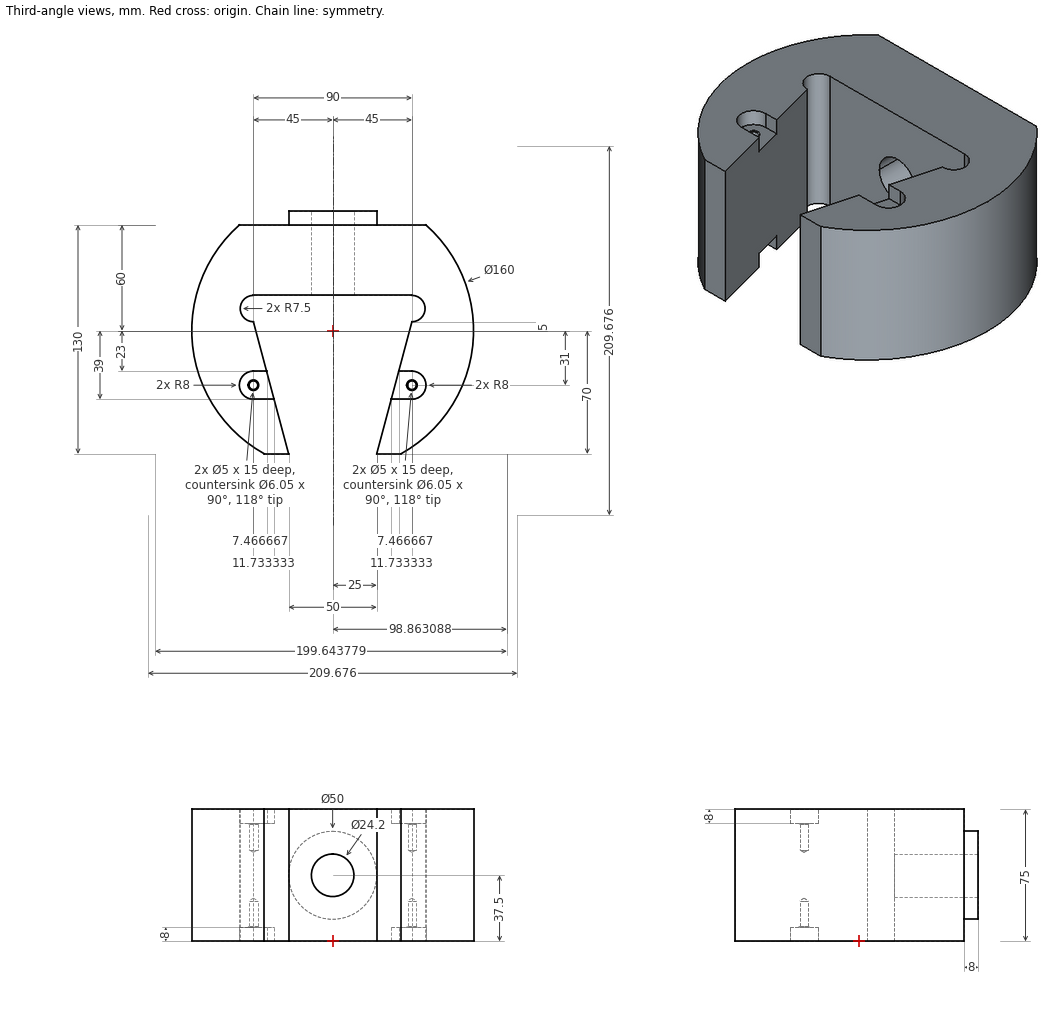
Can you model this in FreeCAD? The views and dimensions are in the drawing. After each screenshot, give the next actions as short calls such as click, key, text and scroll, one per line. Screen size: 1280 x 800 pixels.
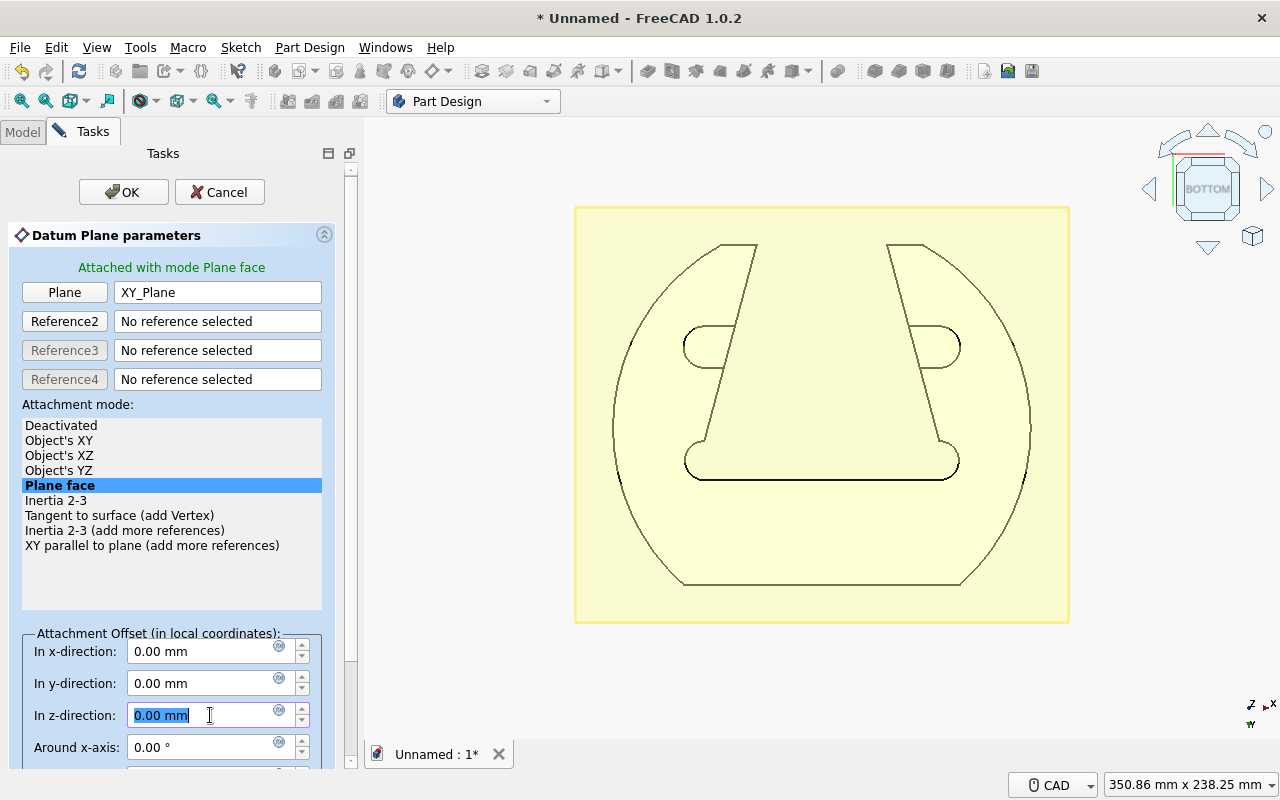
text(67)
key(Tab)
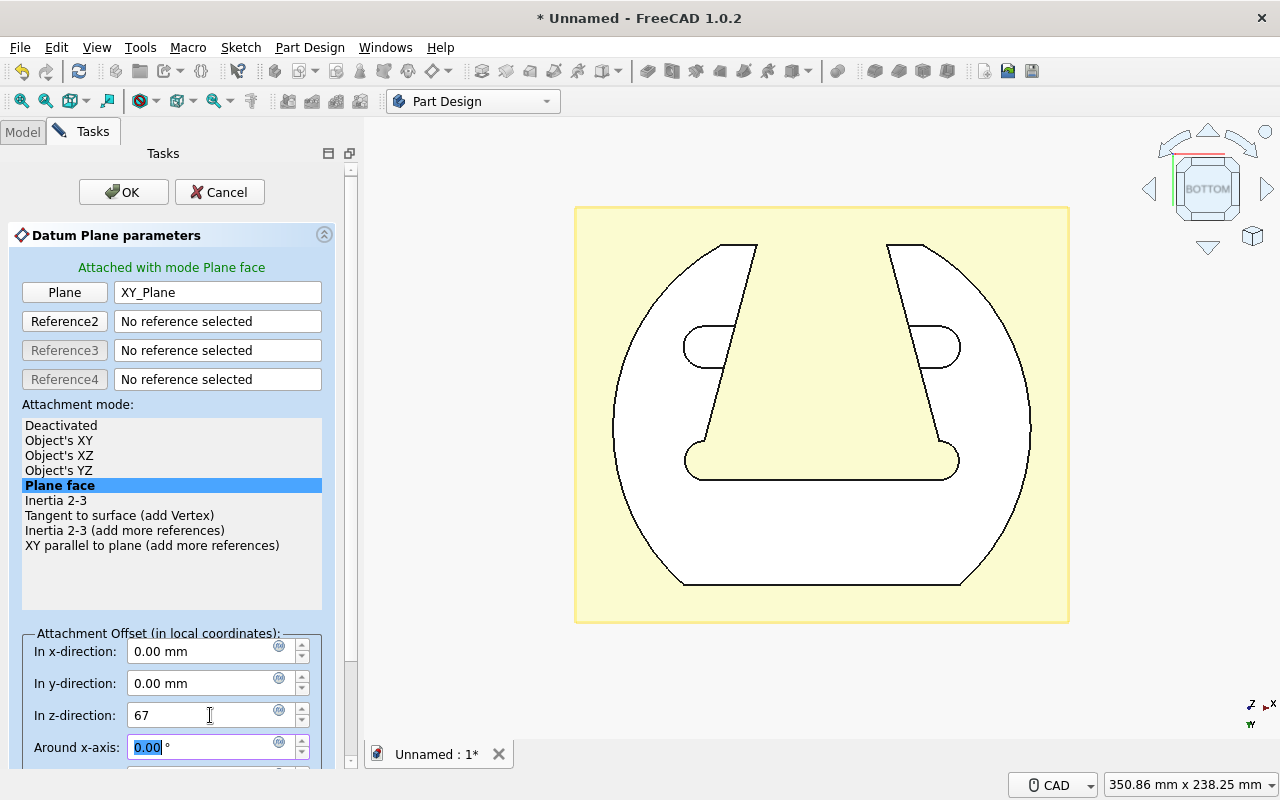
click(124, 192)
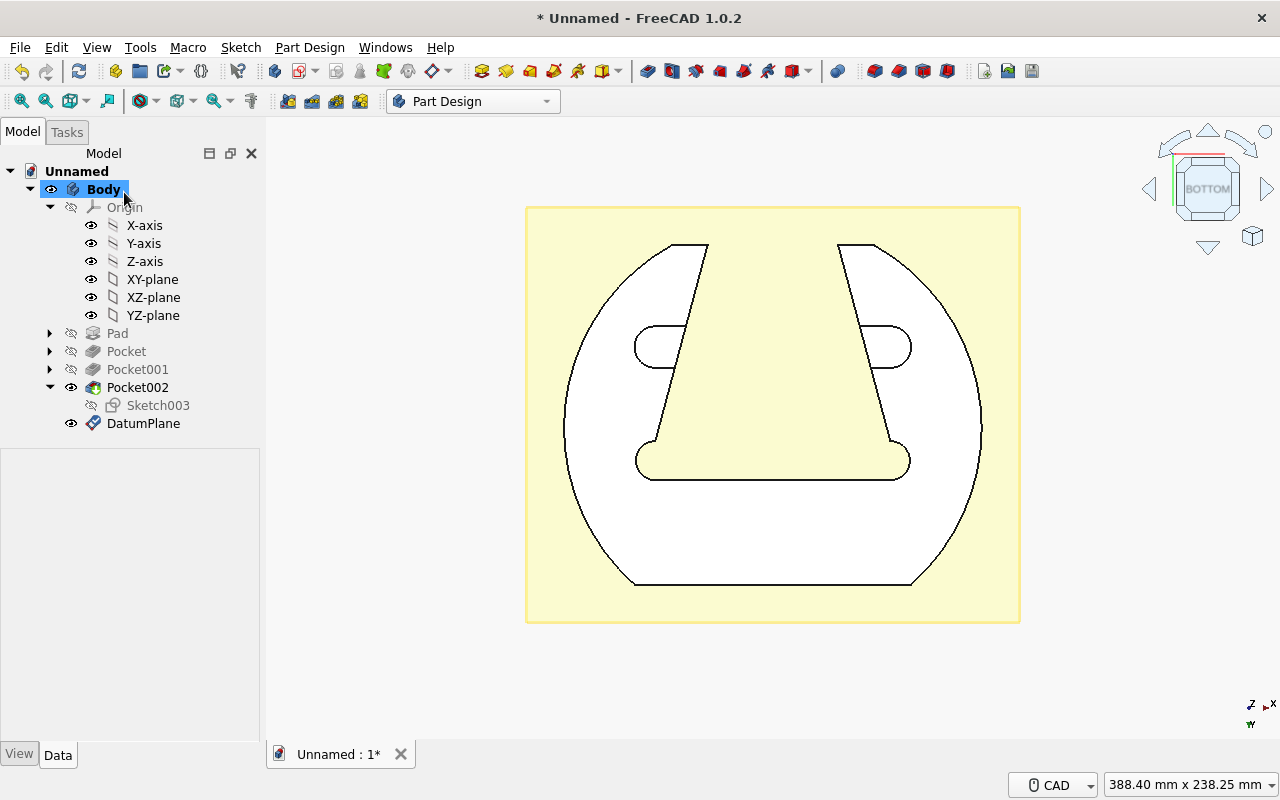
click(116, 423)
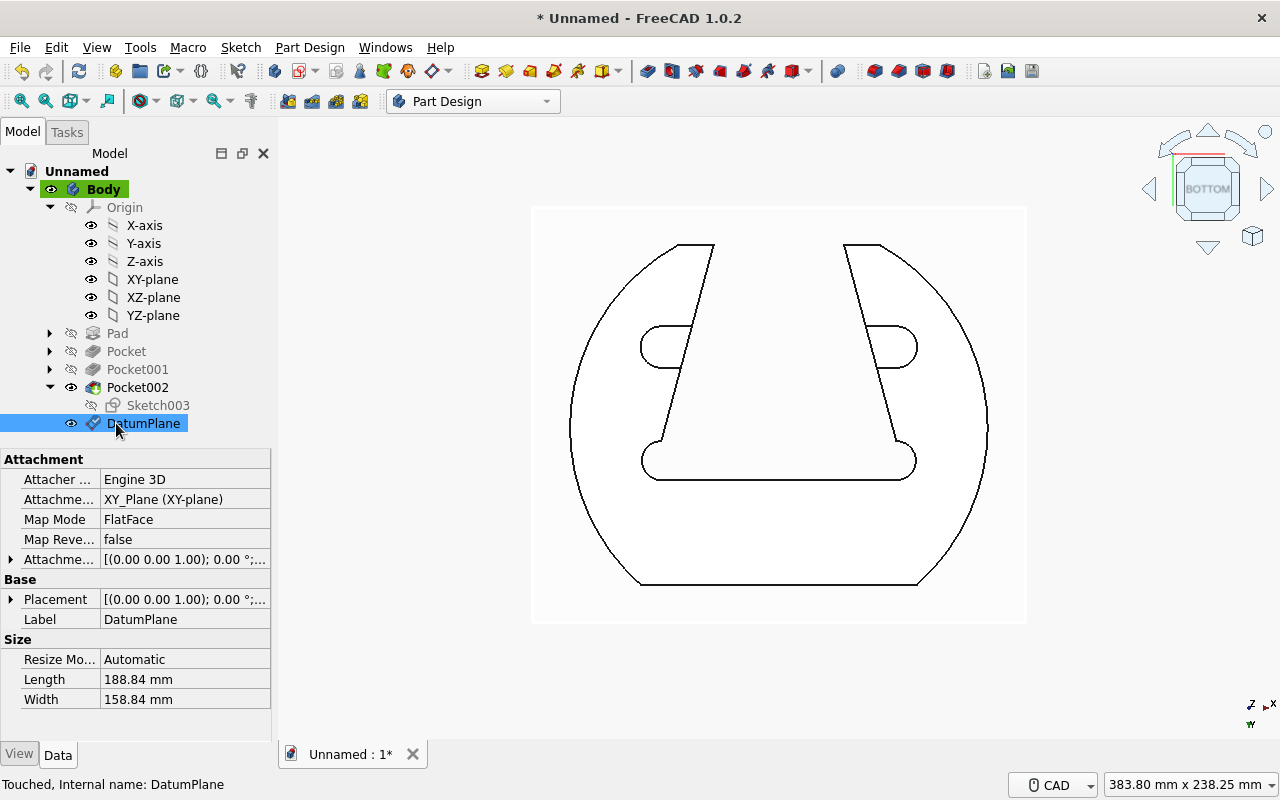
click(300, 72)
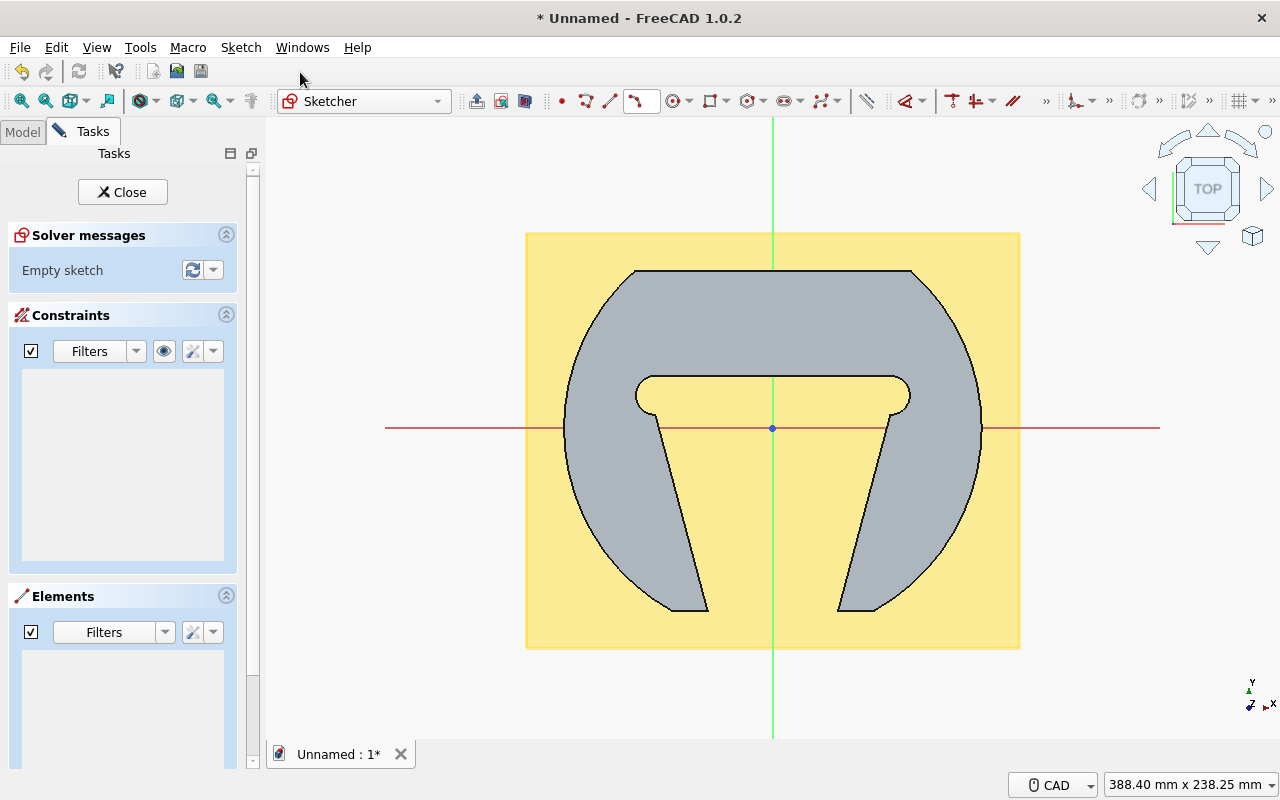
click(526, 102)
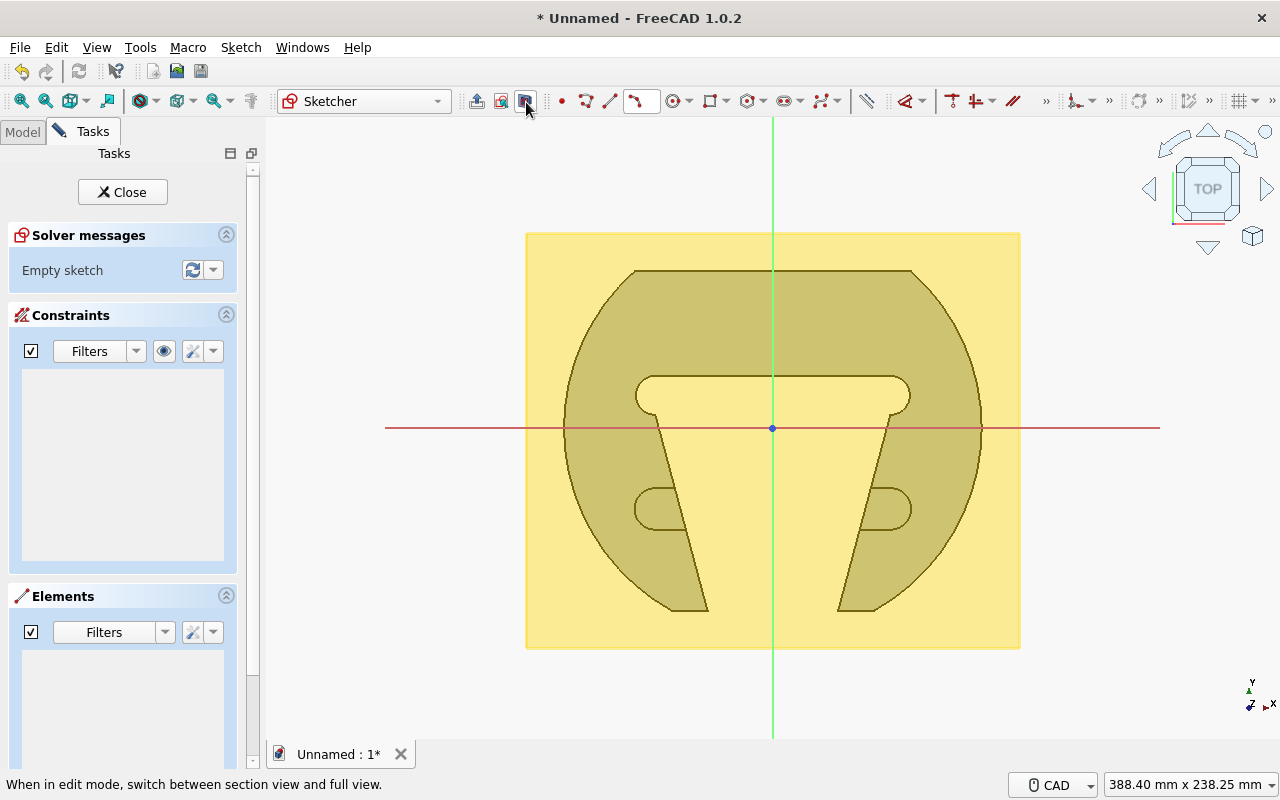
scroll(829, 520, up, 4)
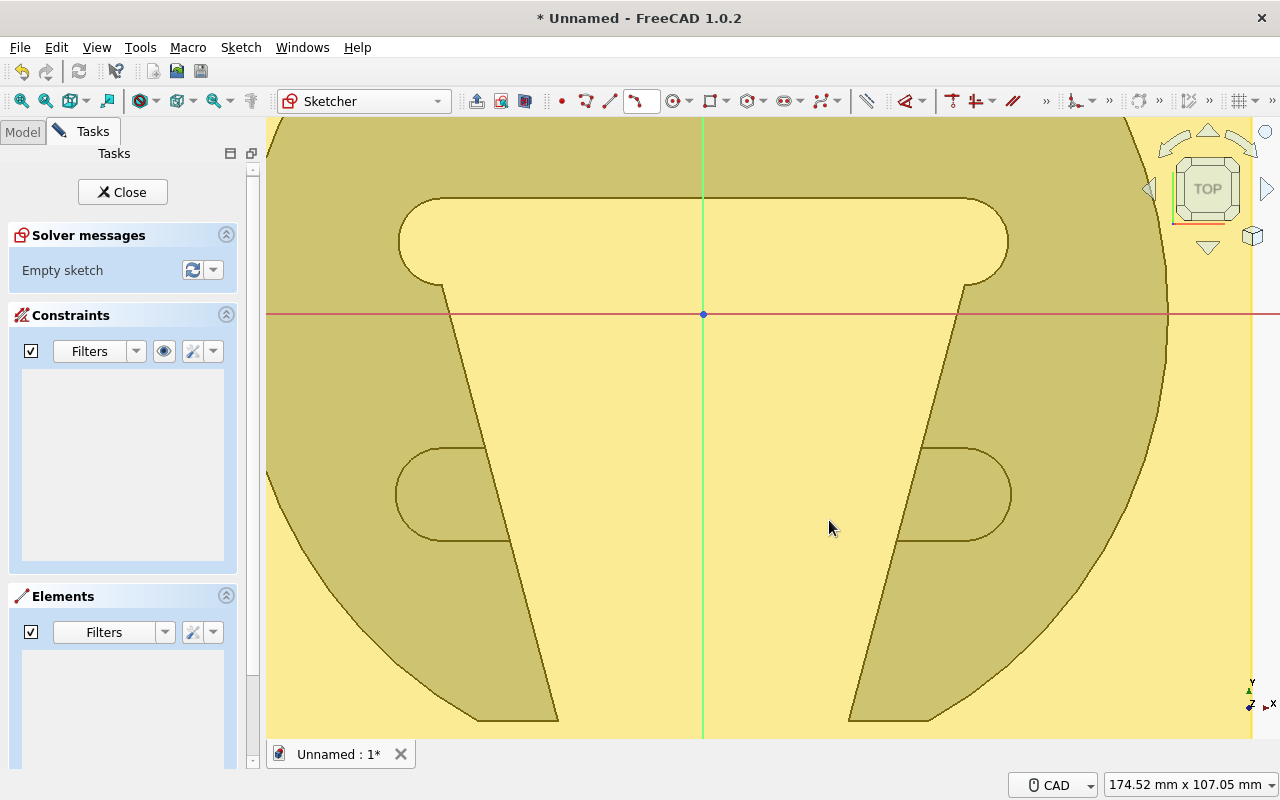
key(g)
key(m)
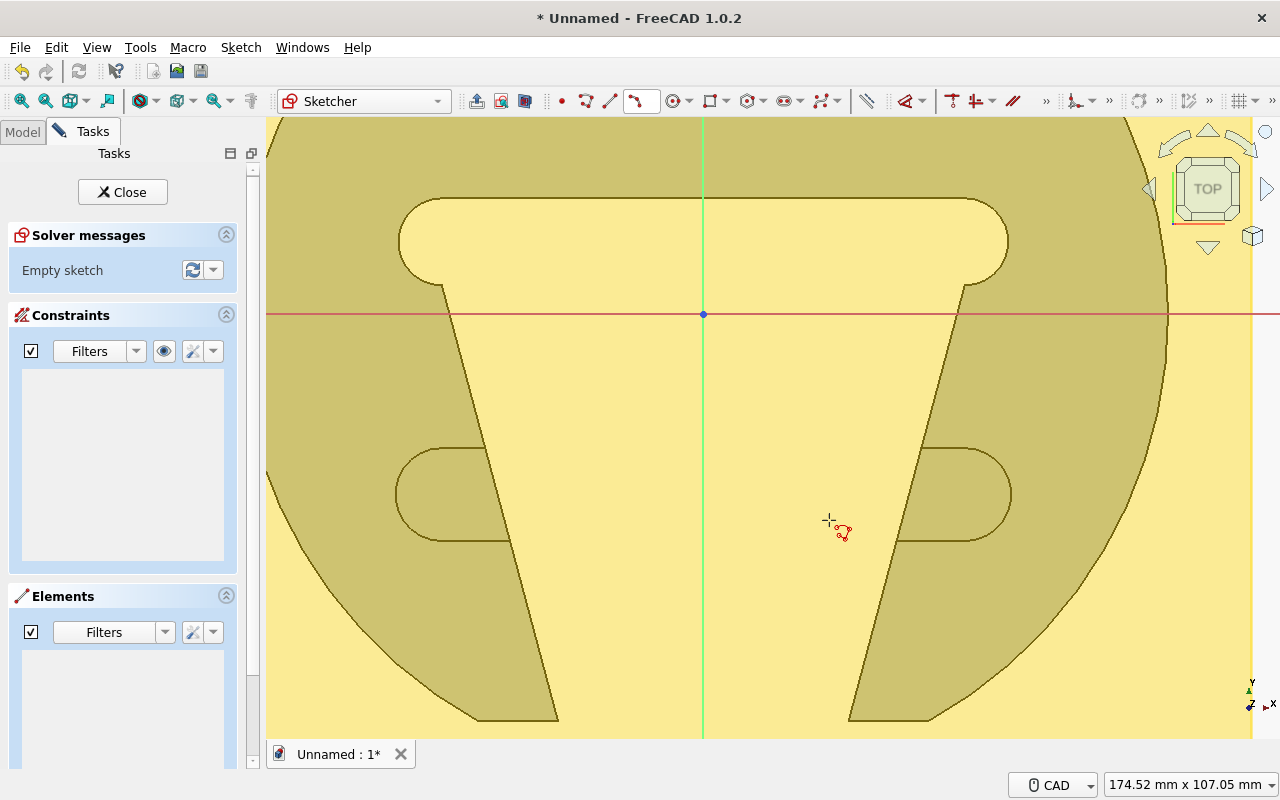
click(442, 448)
click(485, 448)
click(510, 541)
click(442, 541)
right_click(442, 541)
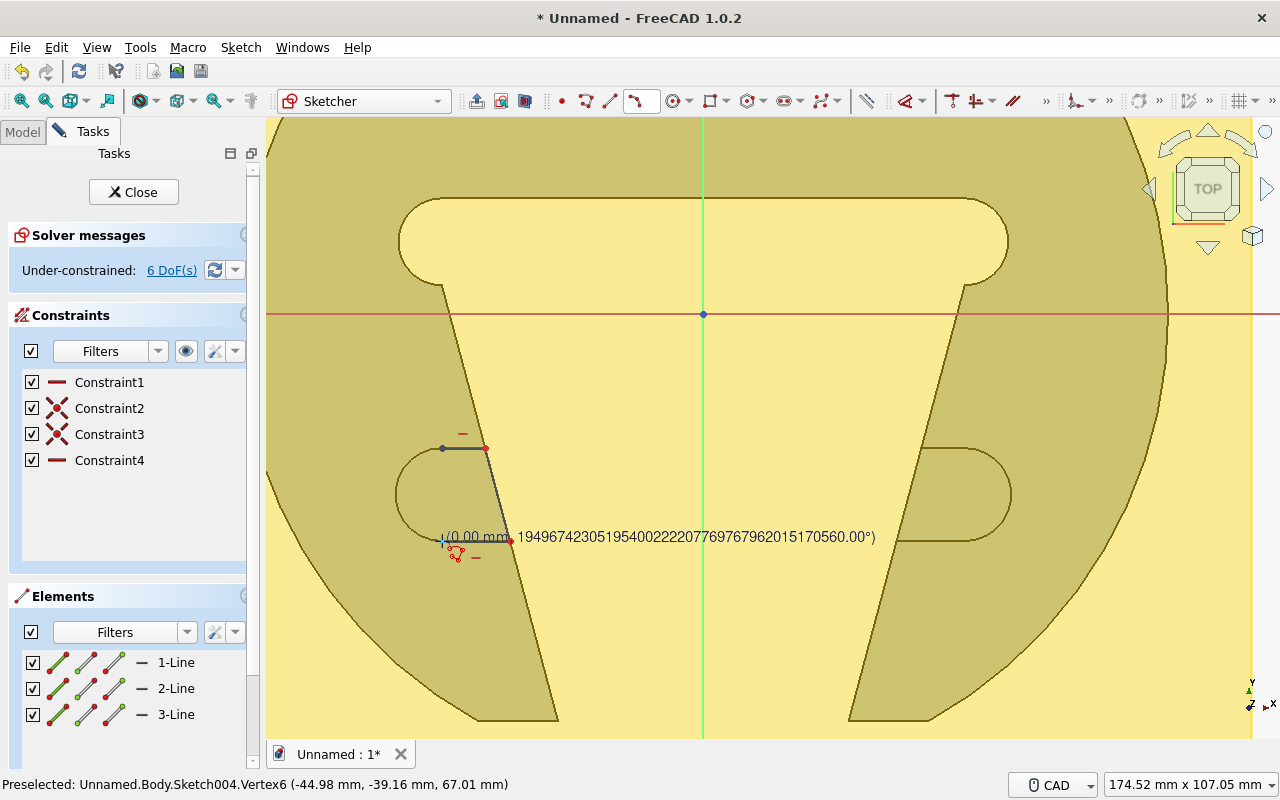
click(636, 102)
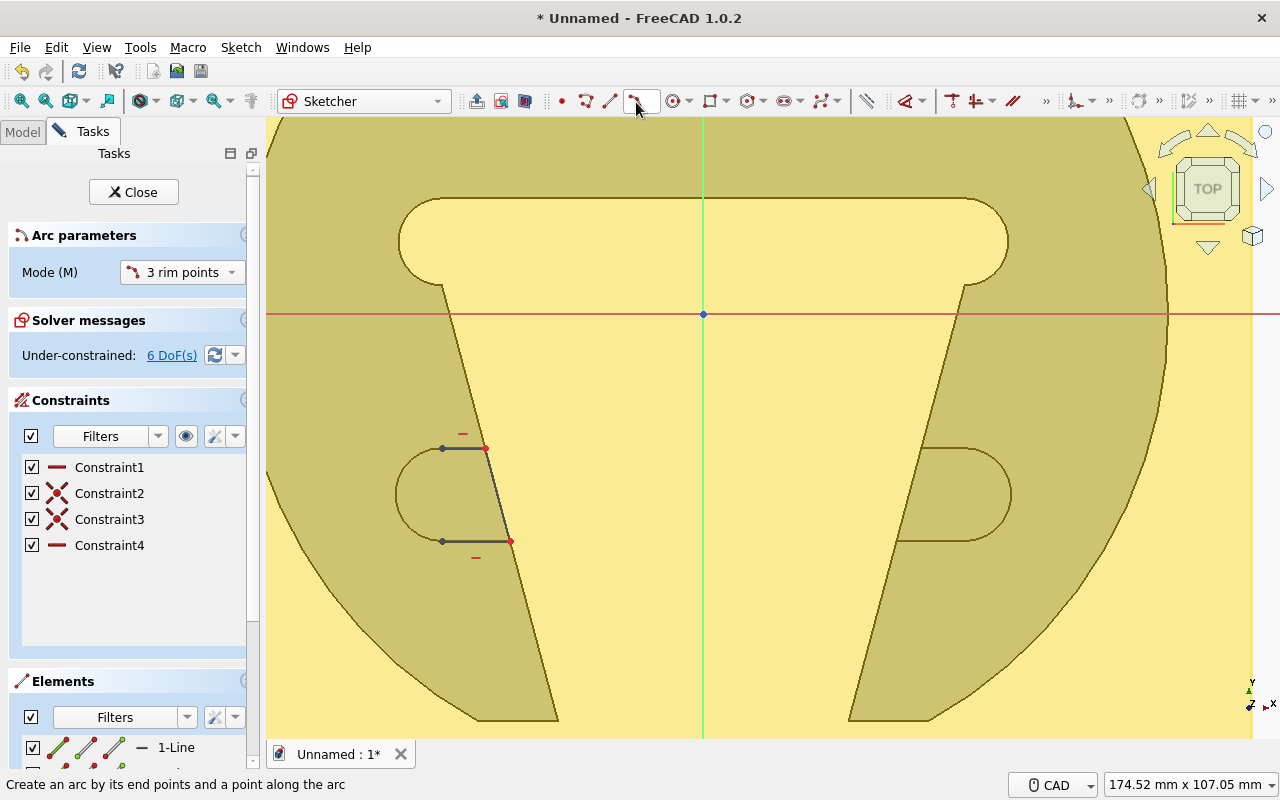
click(442, 542)
click(442, 449)
click(395, 495)